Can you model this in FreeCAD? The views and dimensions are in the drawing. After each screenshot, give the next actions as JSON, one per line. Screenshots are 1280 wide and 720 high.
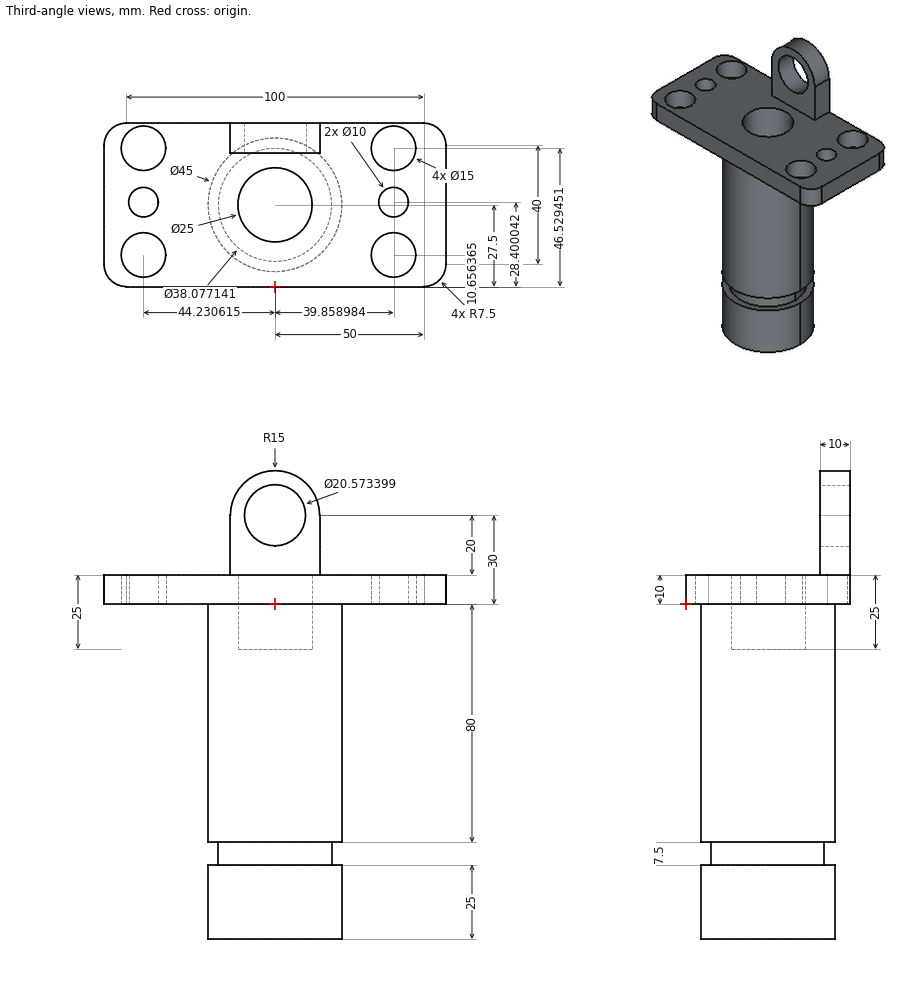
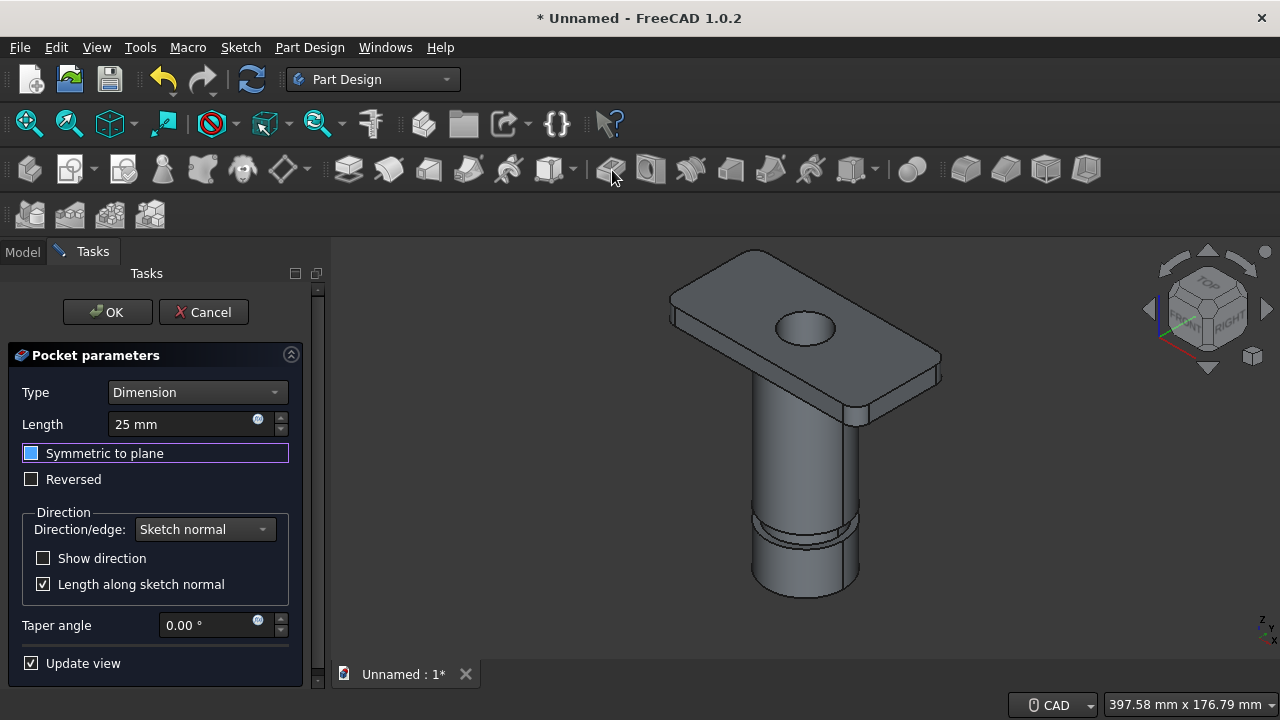
{"action": "left_click", "coordinate": [108, 312]}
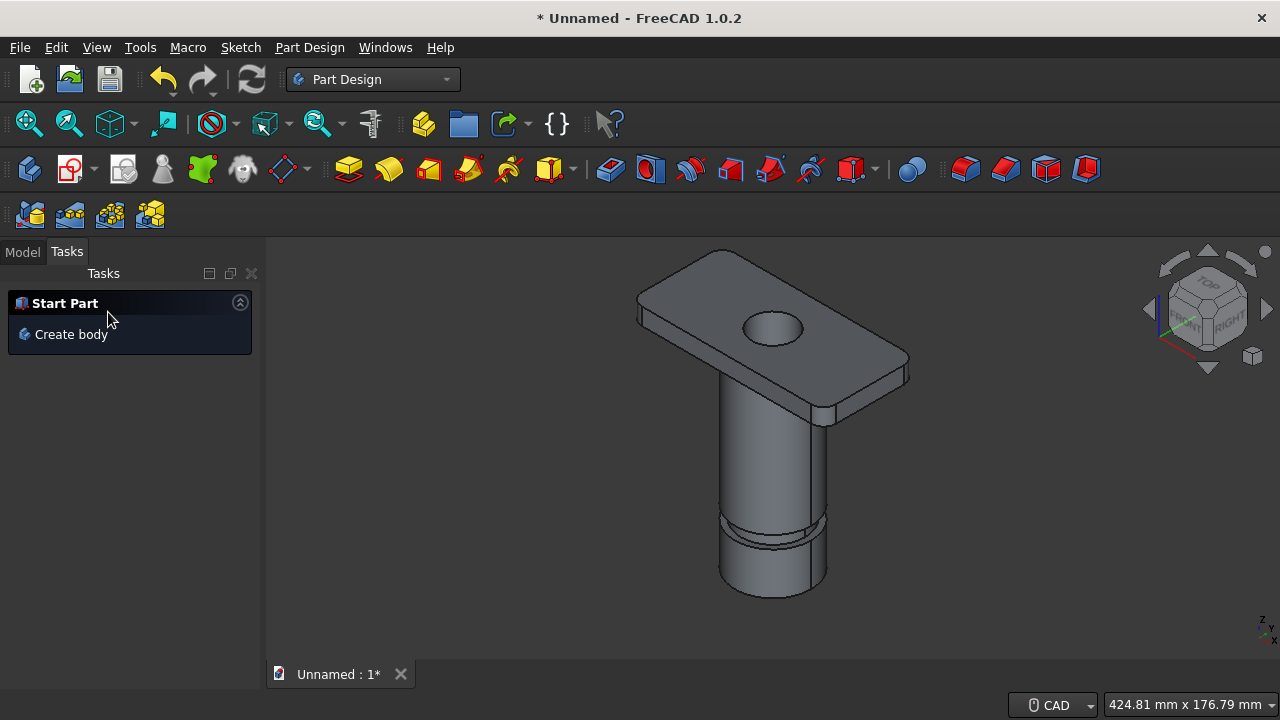
{"action": "left_click", "coordinate": [718, 296]}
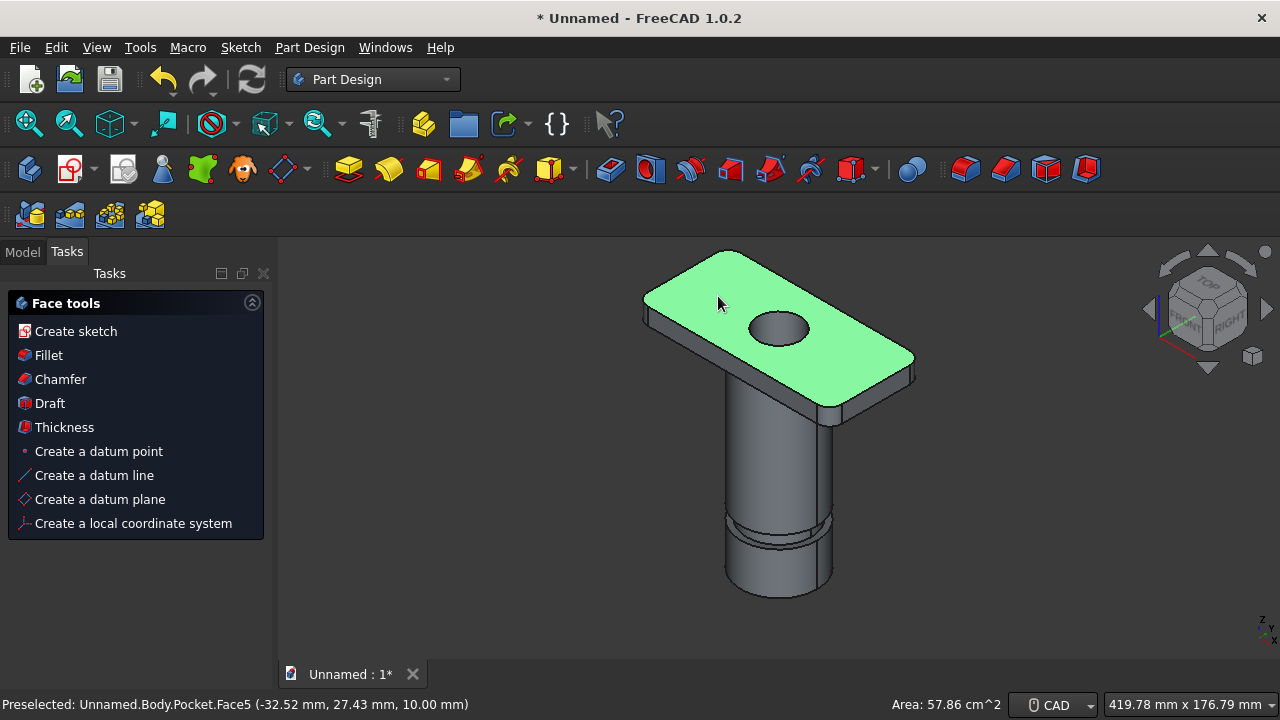
{"action": "left_click", "coordinate": [70, 170]}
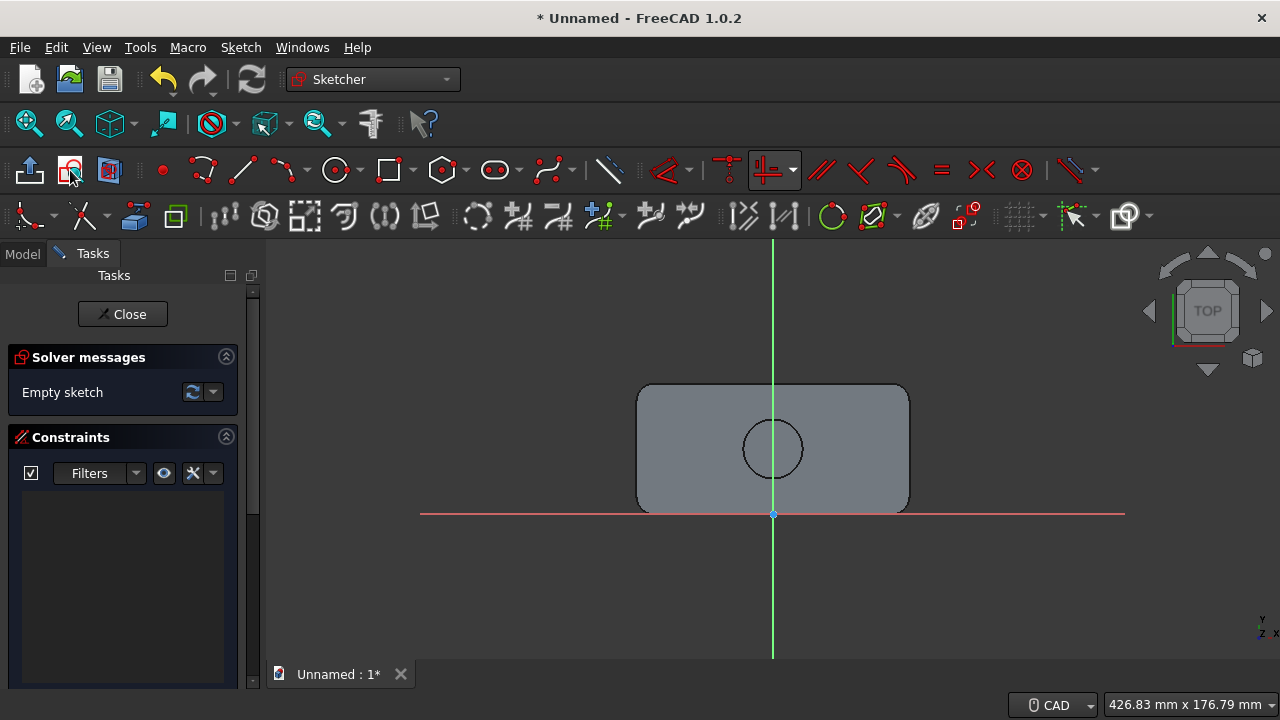
{"action": "scroll", "coordinate": [845, 452], "scroll_direction": "up", "scroll_amount": 3}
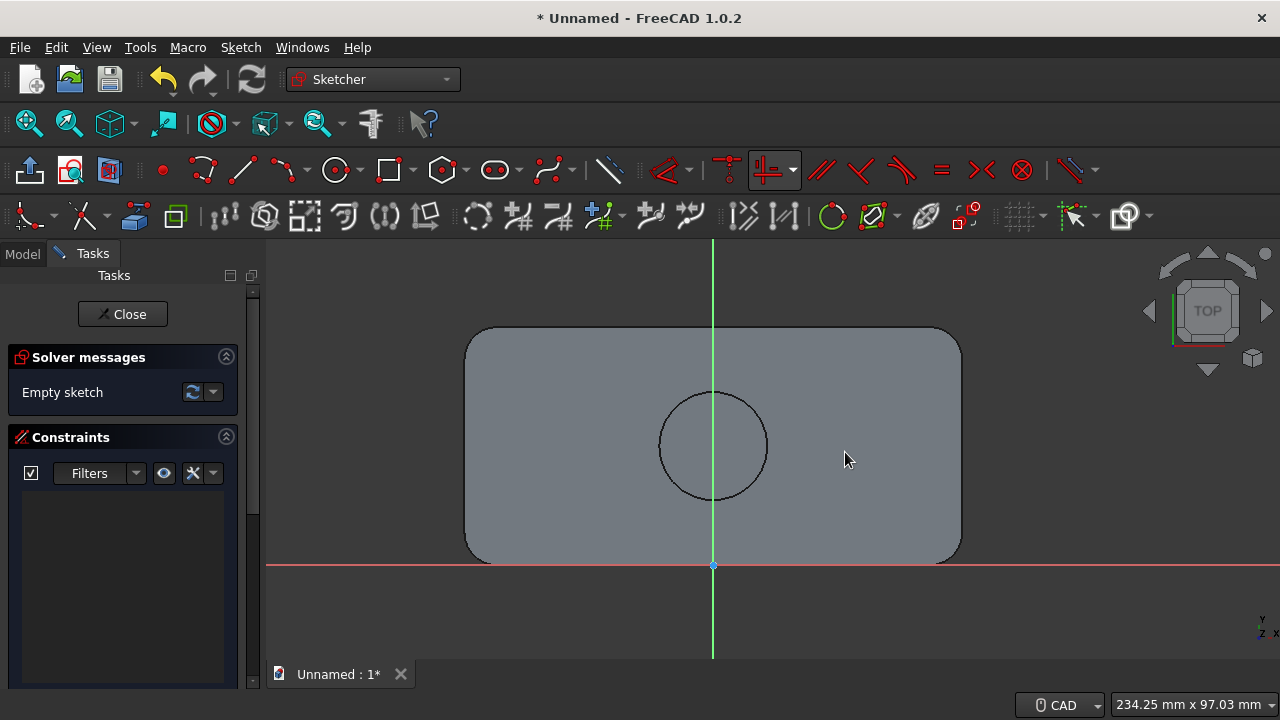
{"action": "left_click", "coordinate": [336, 170]}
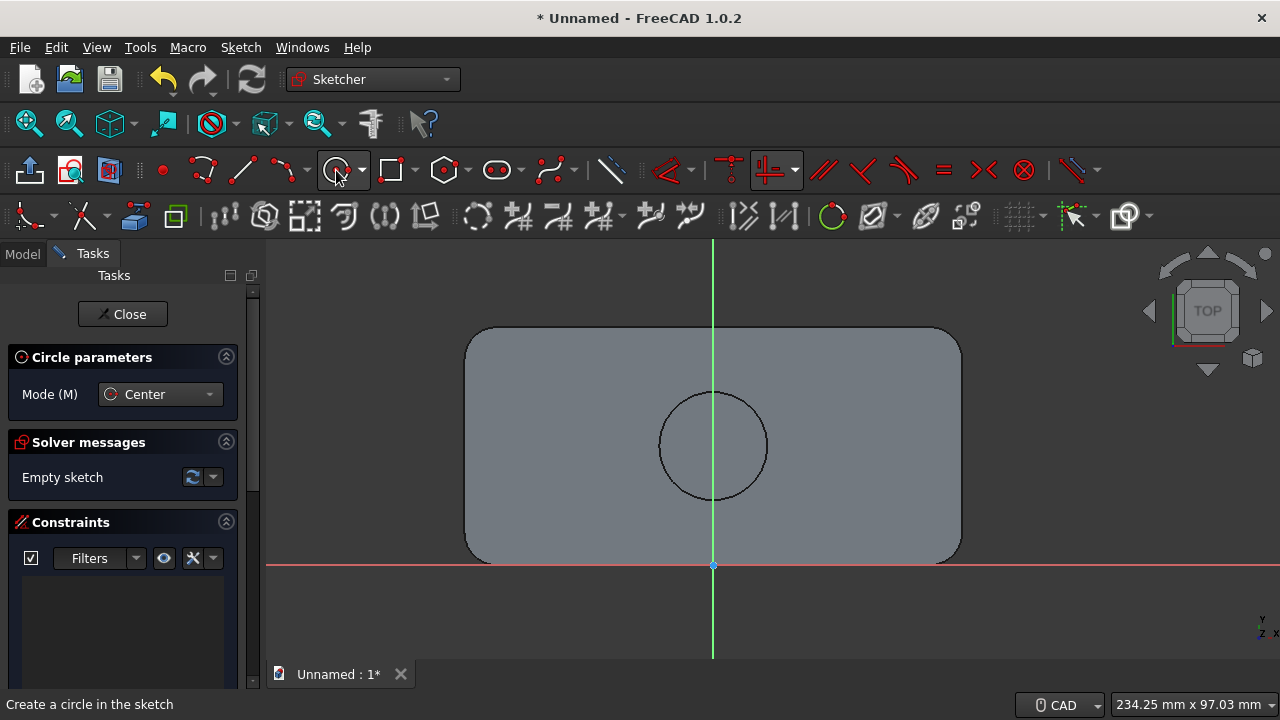
{"action": "left_click", "coordinate": [886, 364]}
{"action": "left_click", "coordinate": [909, 341]}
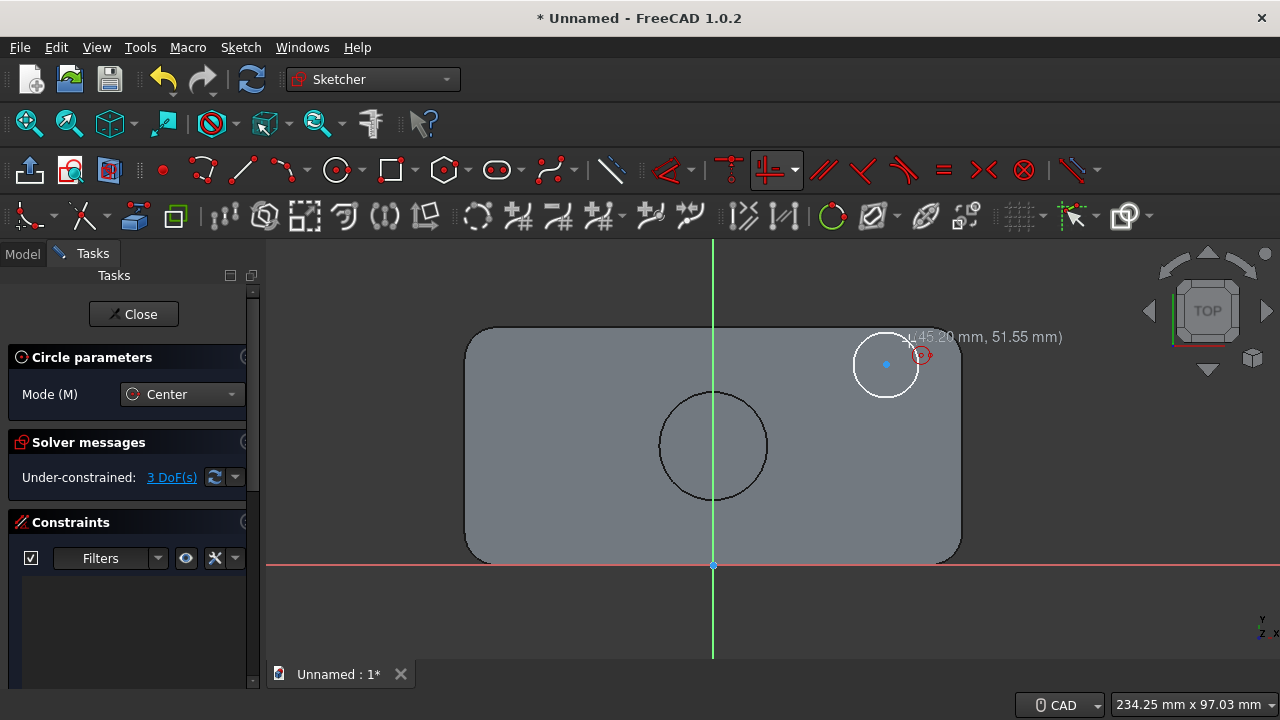
{"action": "left_click", "coordinate": [886, 442]}
{"action": "left_click", "coordinate": [901, 427]}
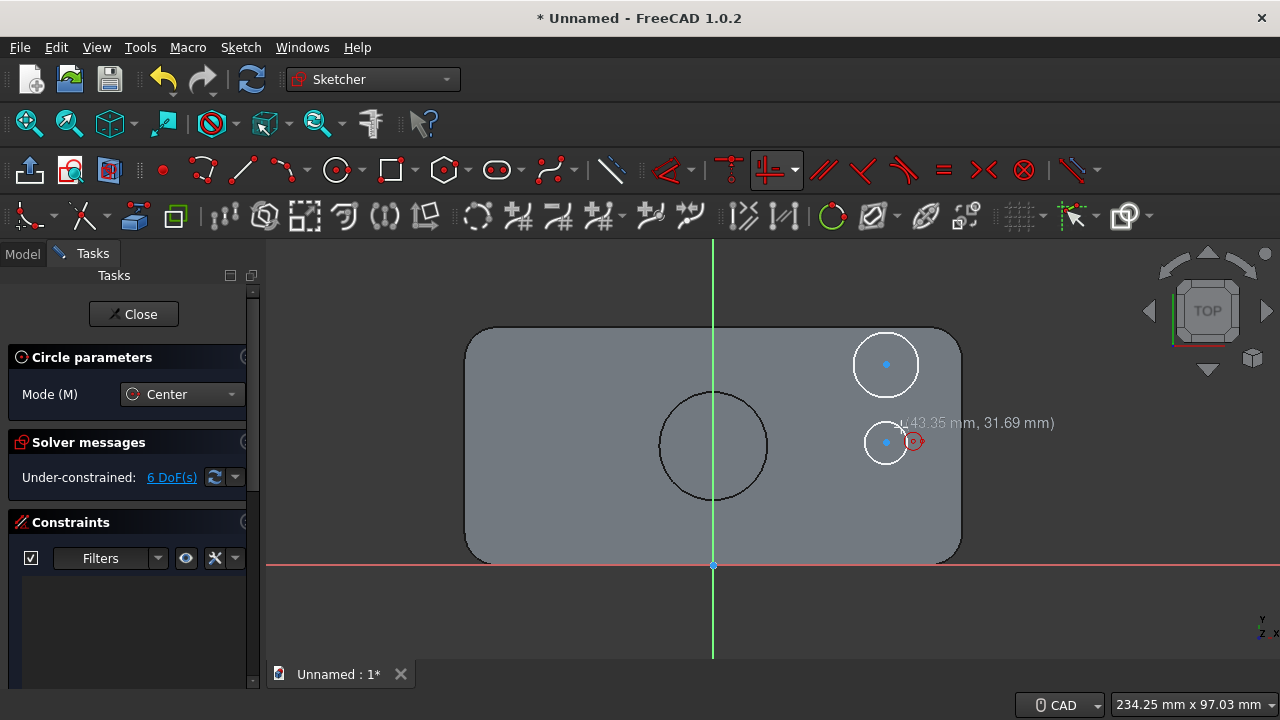
{"action": "left_click", "coordinate": [886, 519]}
{"action": "left_click", "coordinate": [909, 496]}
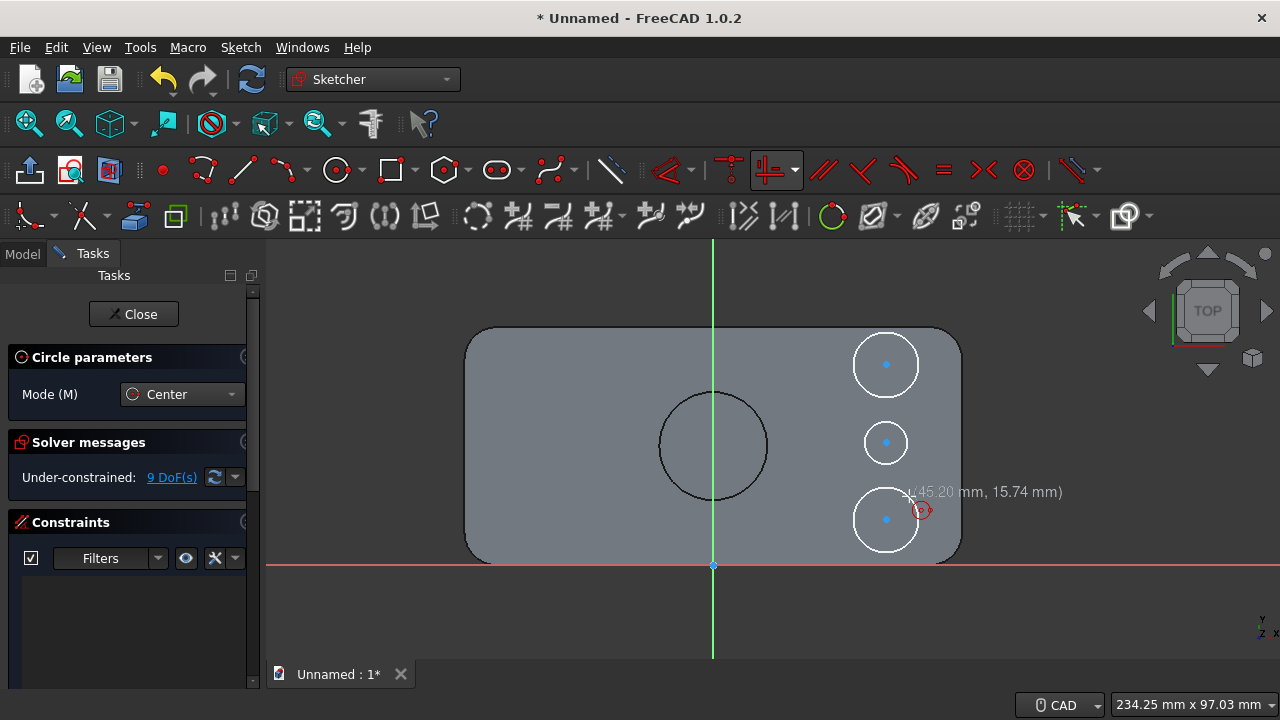
{"action": "left_click", "coordinate": [522, 519]}
{"action": "left_click", "coordinate": [545, 496]}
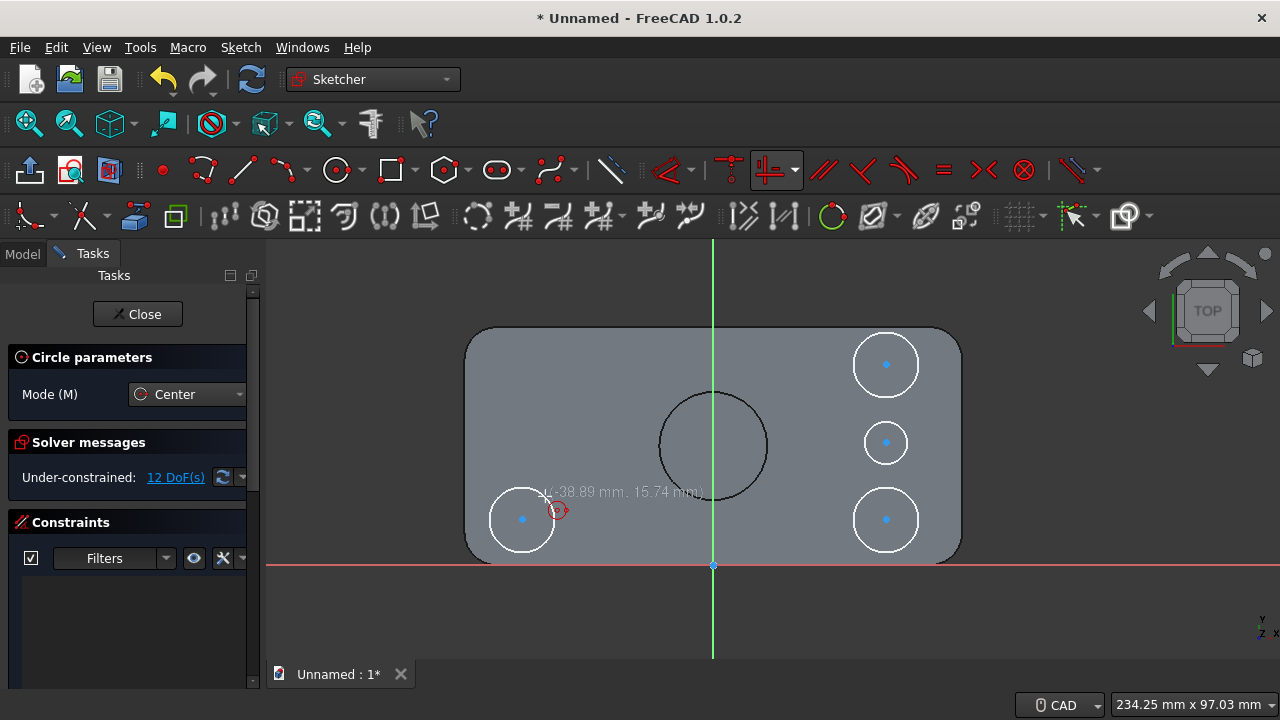
{"action": "left_click", "coordinate": [522, 442]}
{"action": "left_click", "coordinate": [537, 427]}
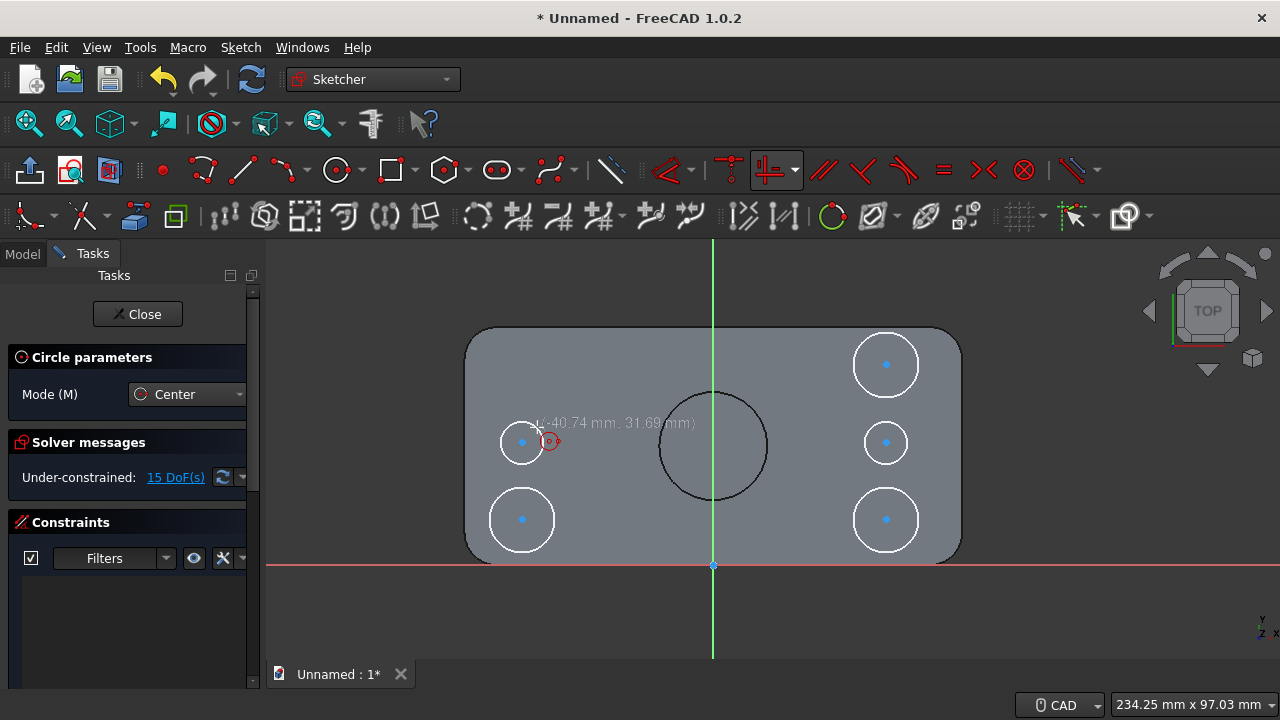
{"action": "left_click", "coordinate": [522, 364]}
{"action": "left_click", "coordinate": [545, 341]}
{"action": "key", "text": "Escape"}